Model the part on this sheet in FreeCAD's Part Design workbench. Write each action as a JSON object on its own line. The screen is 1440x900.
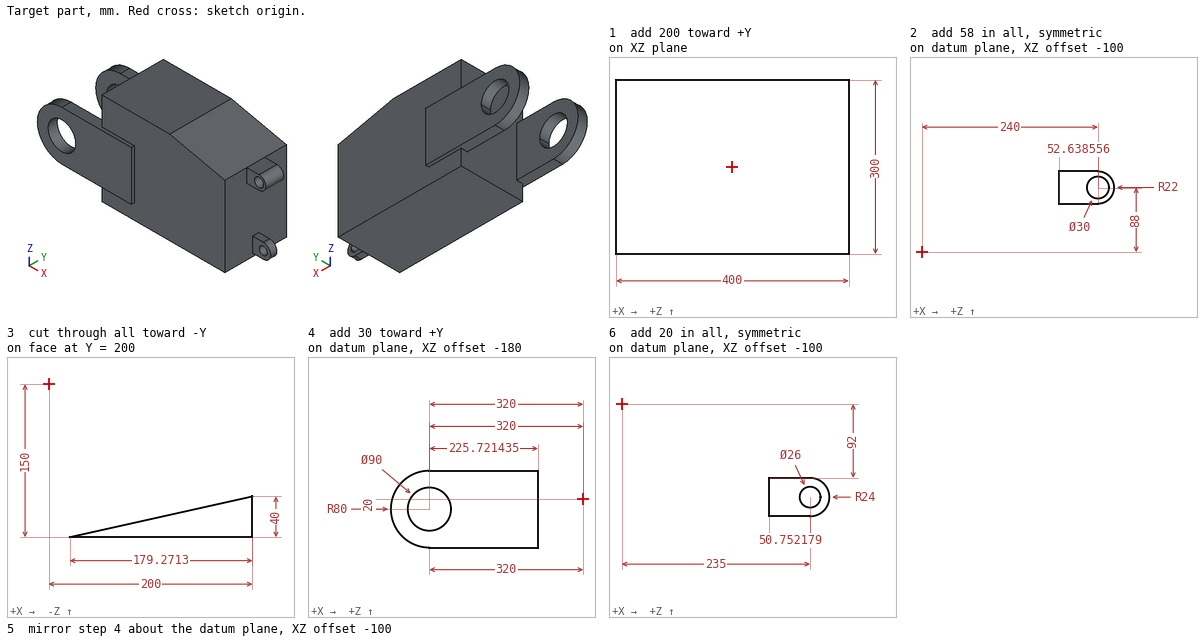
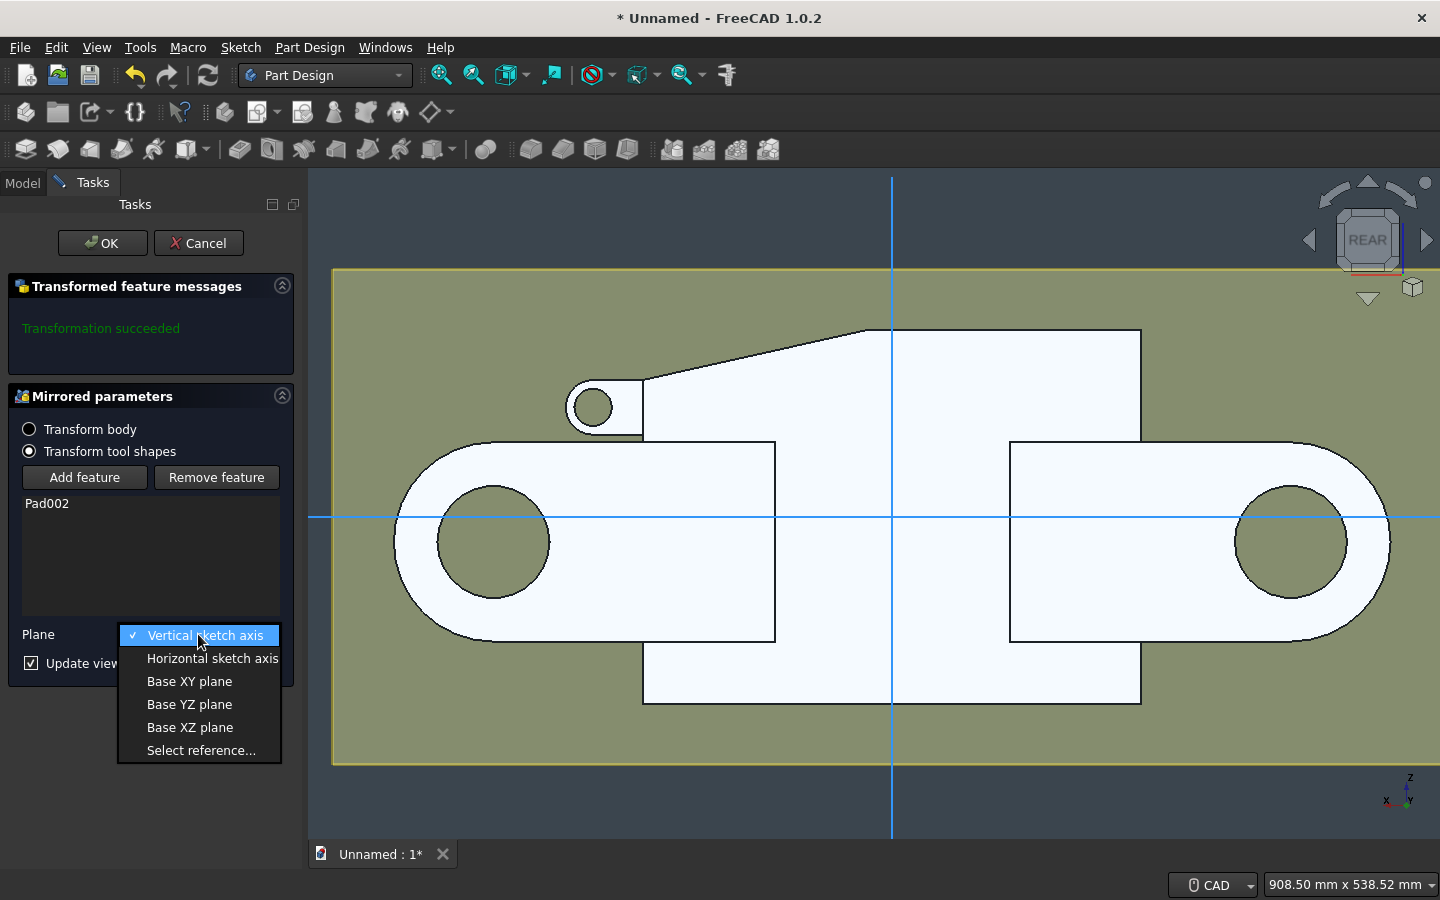
{"action": "left_click", "coordinate": [198, 750]}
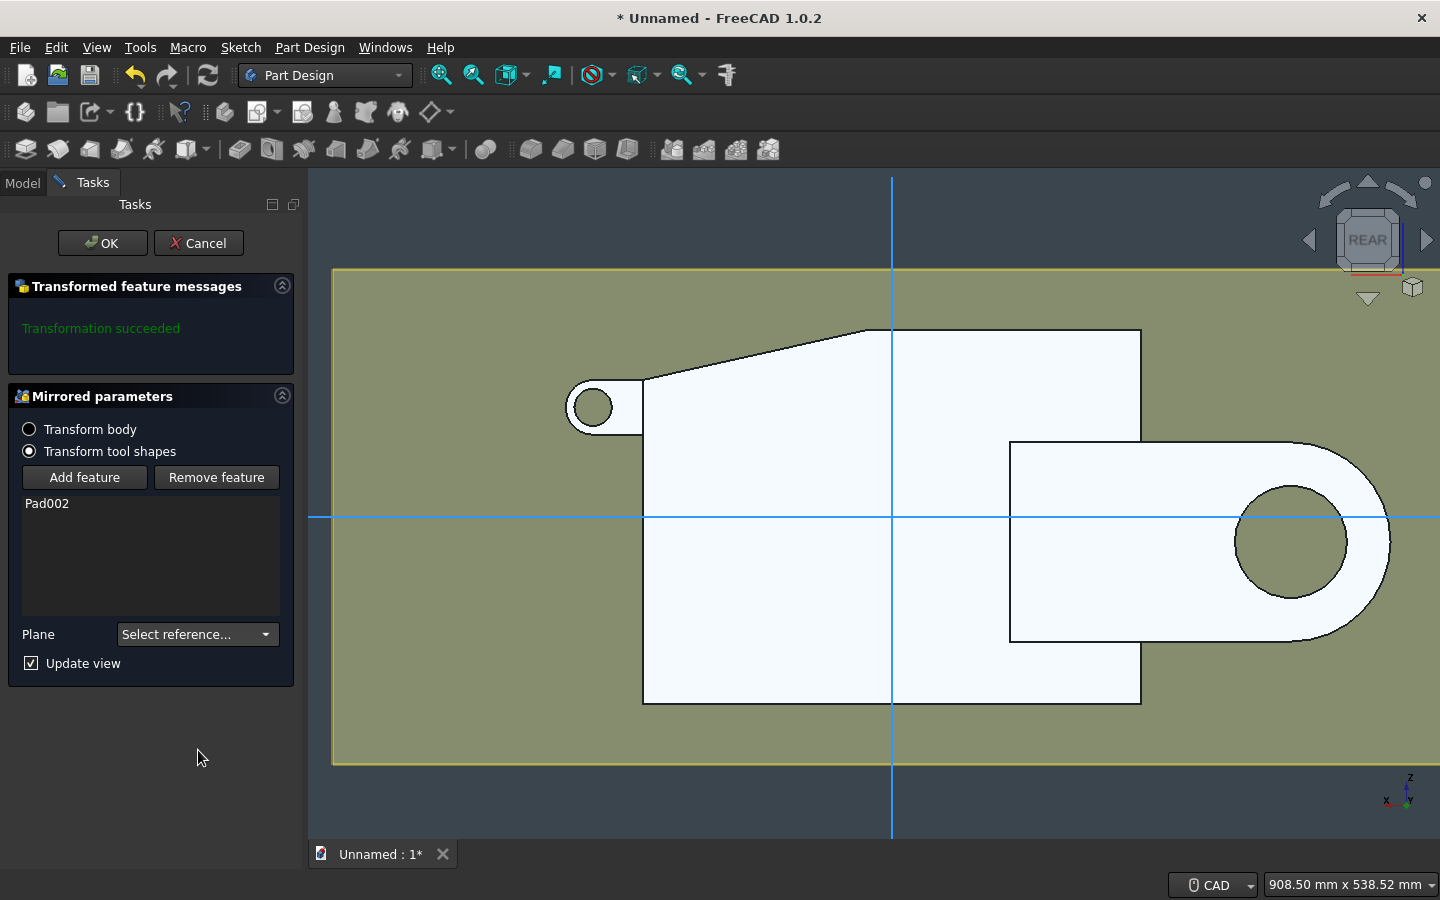
{"action": "left_click", "coordinate": [23, 182]}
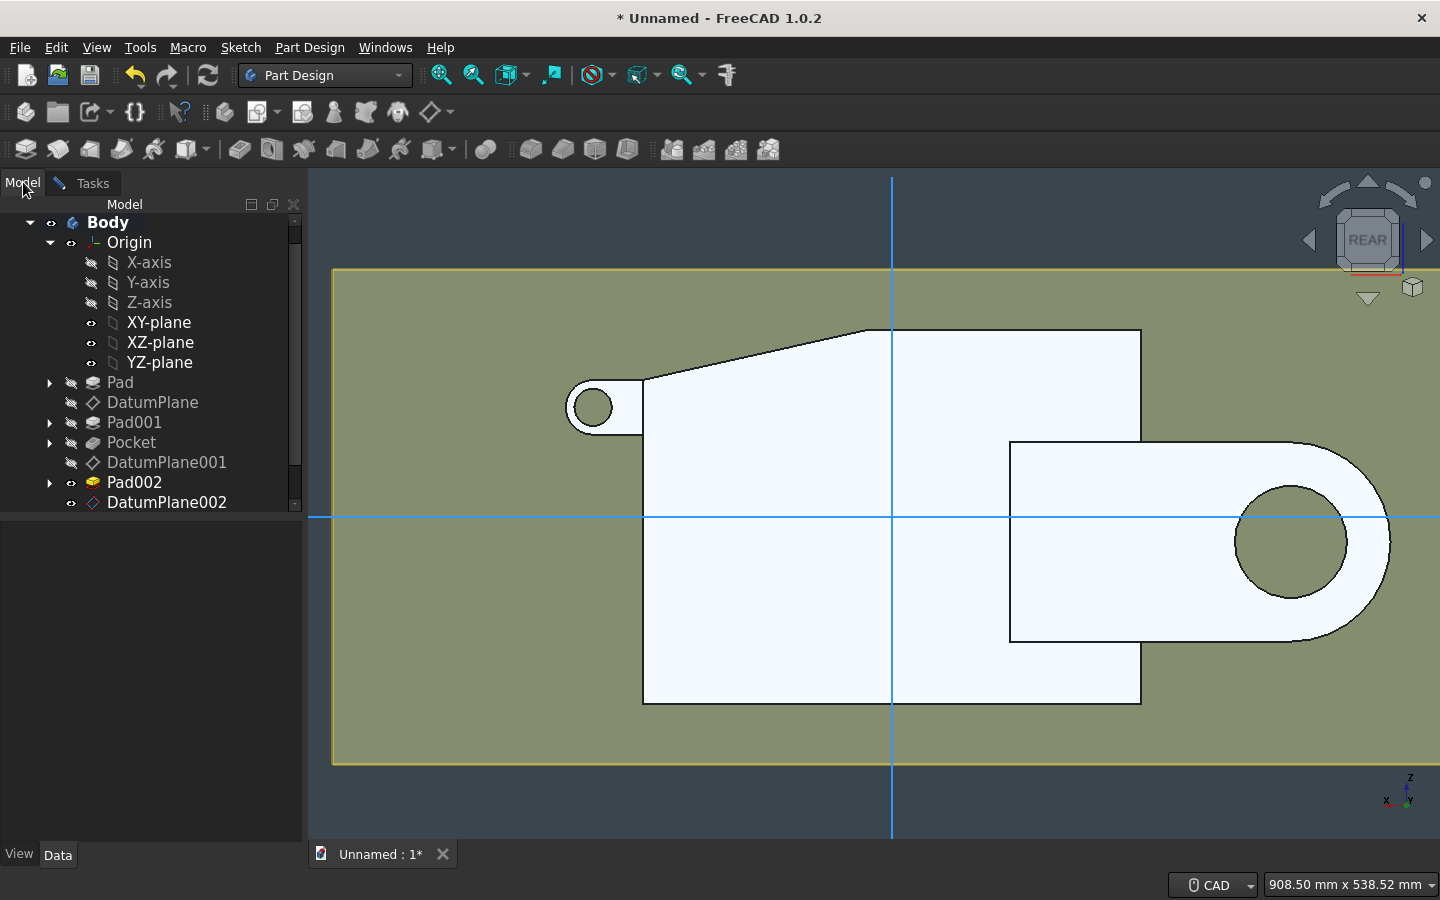
{"action": "left_click", "coordinate": [116, 503]}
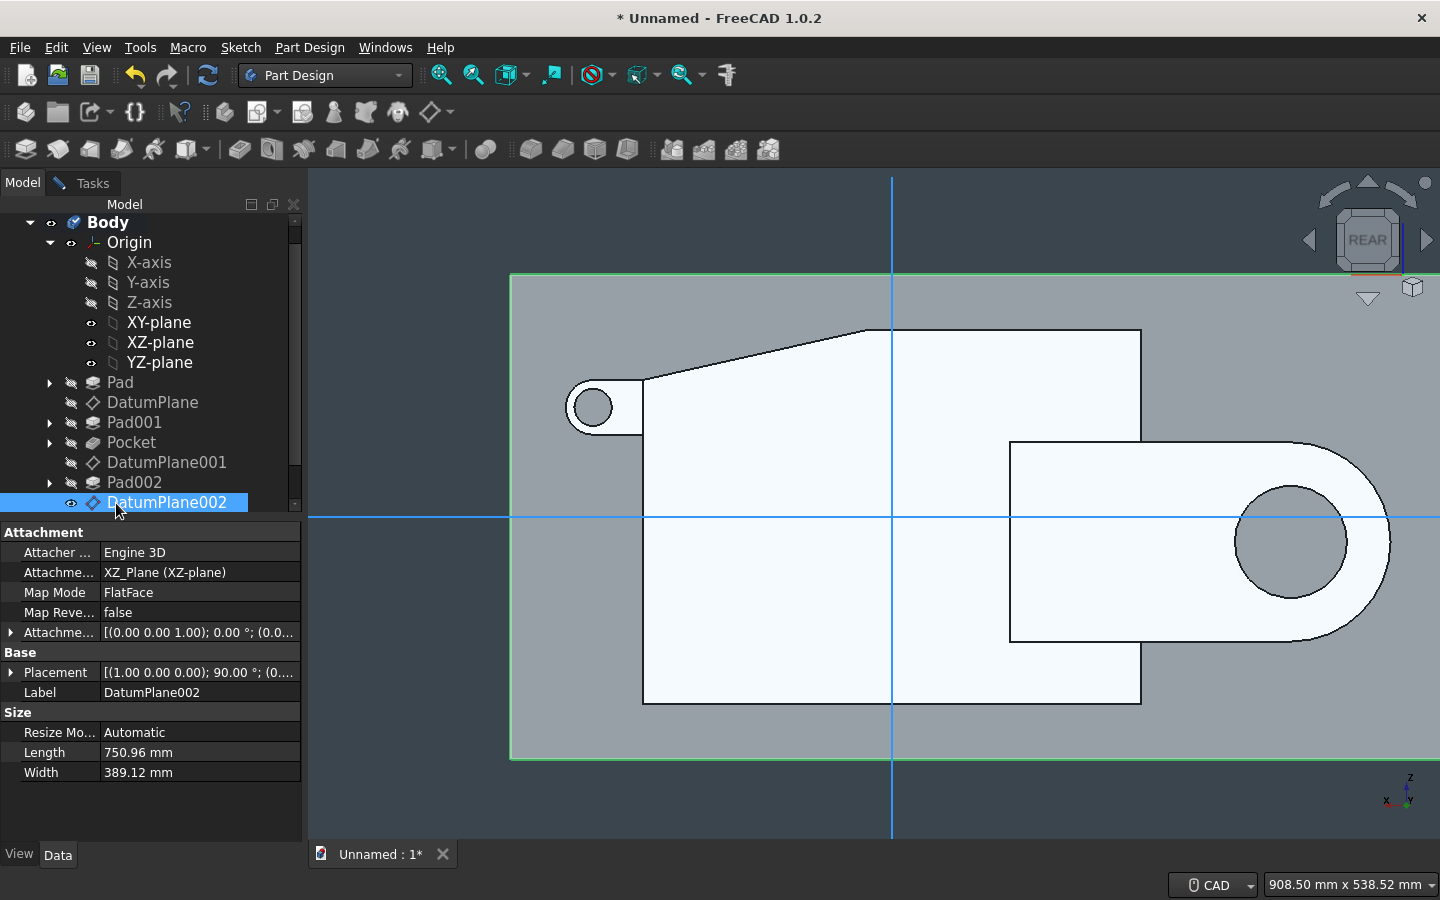
{"action": "left_click", "coordinate": [84, 182]}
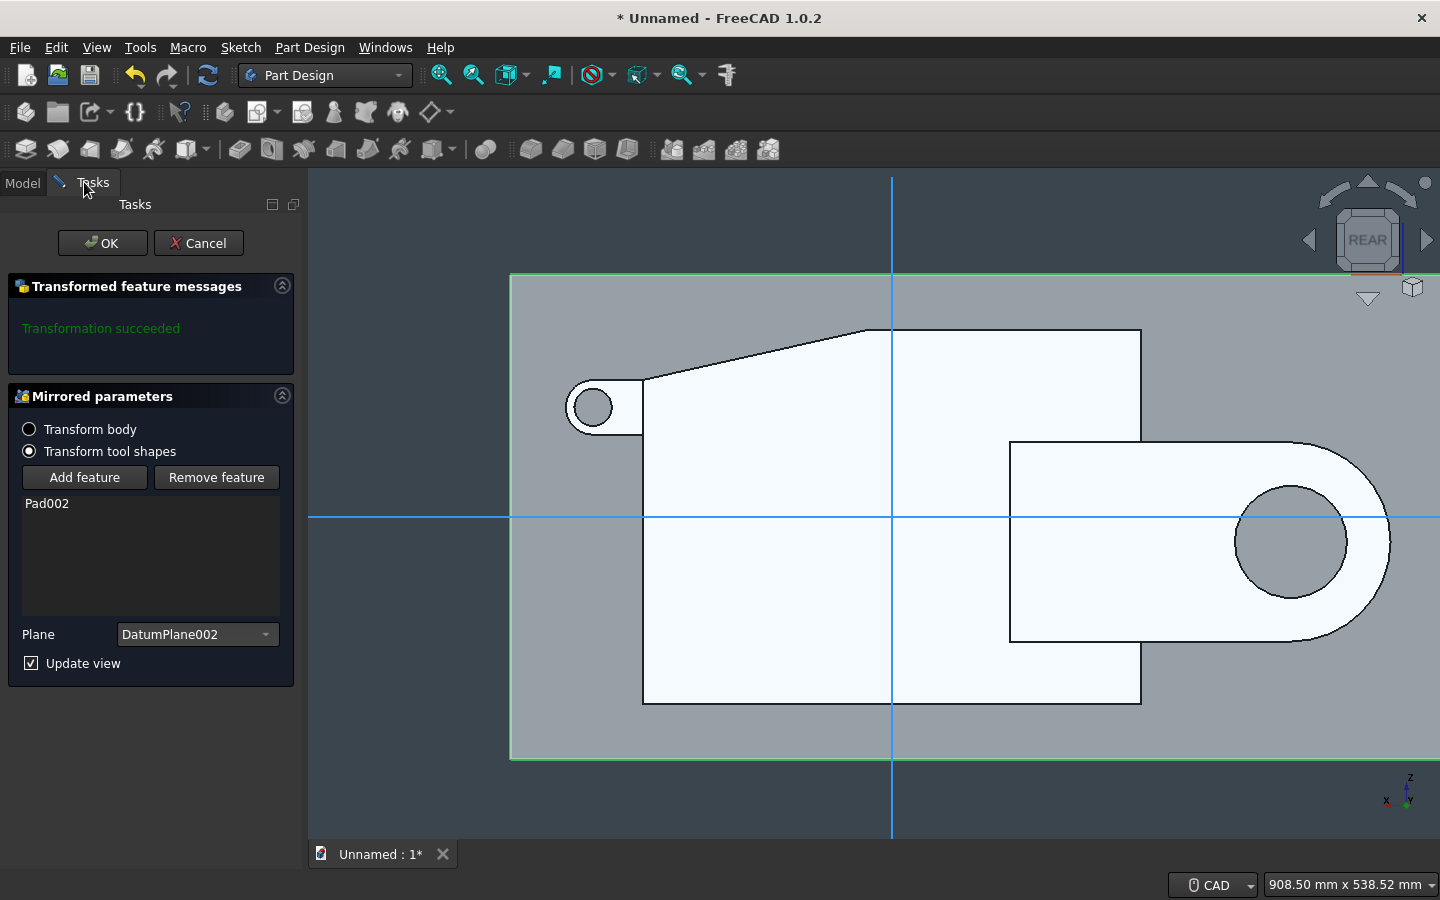
{"action": "left_click", "coordinate": [103, 243]}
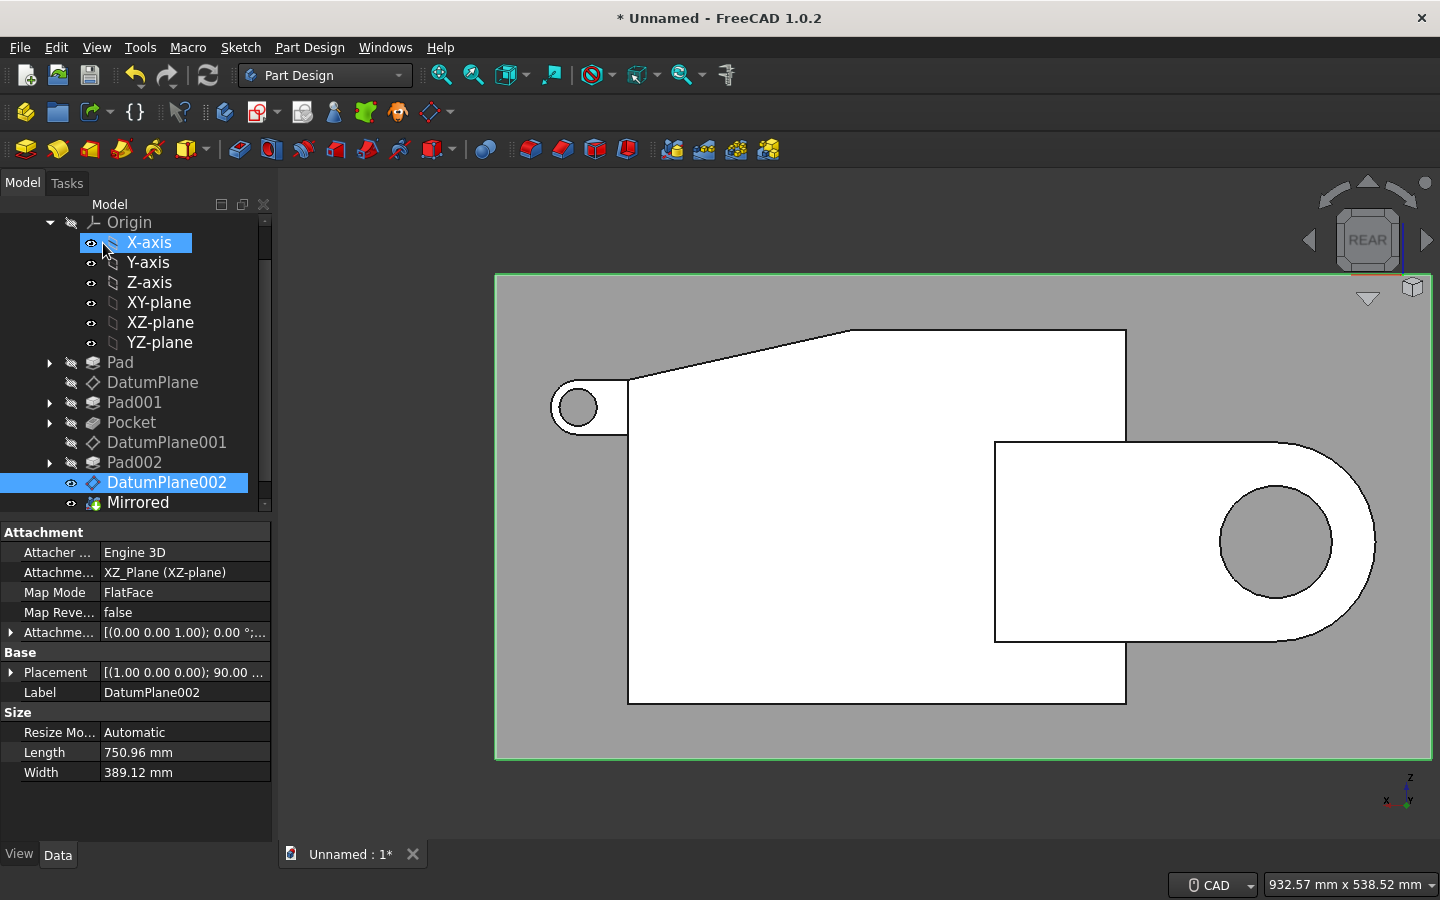
{"action": "left_click", "coordinate": [116, 483]}
{"action": "key", "text": "space"}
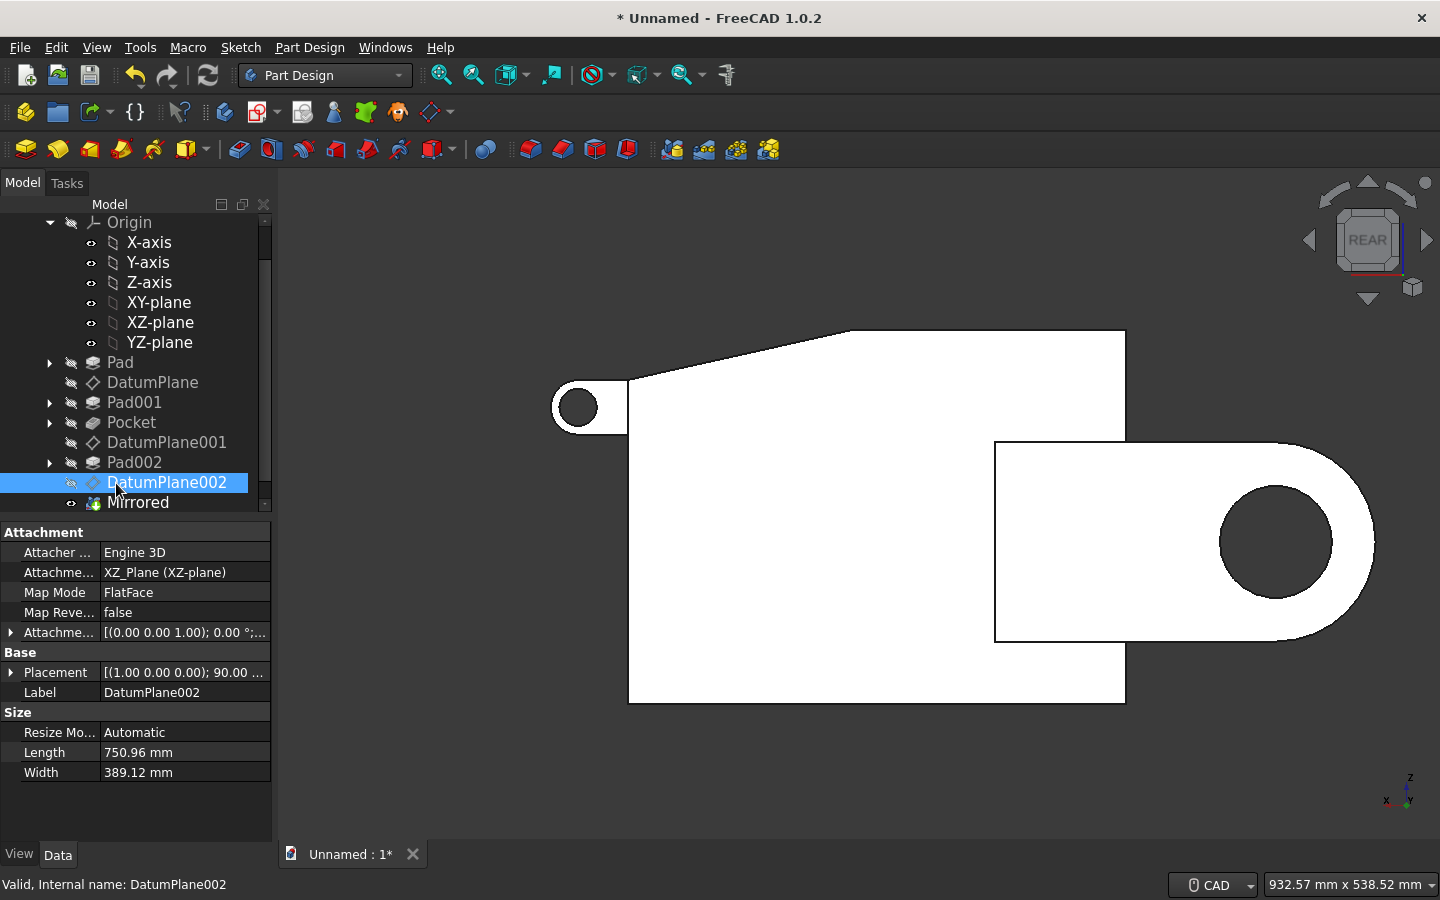
{"action": "left_click", "coordinate": [136, 323]}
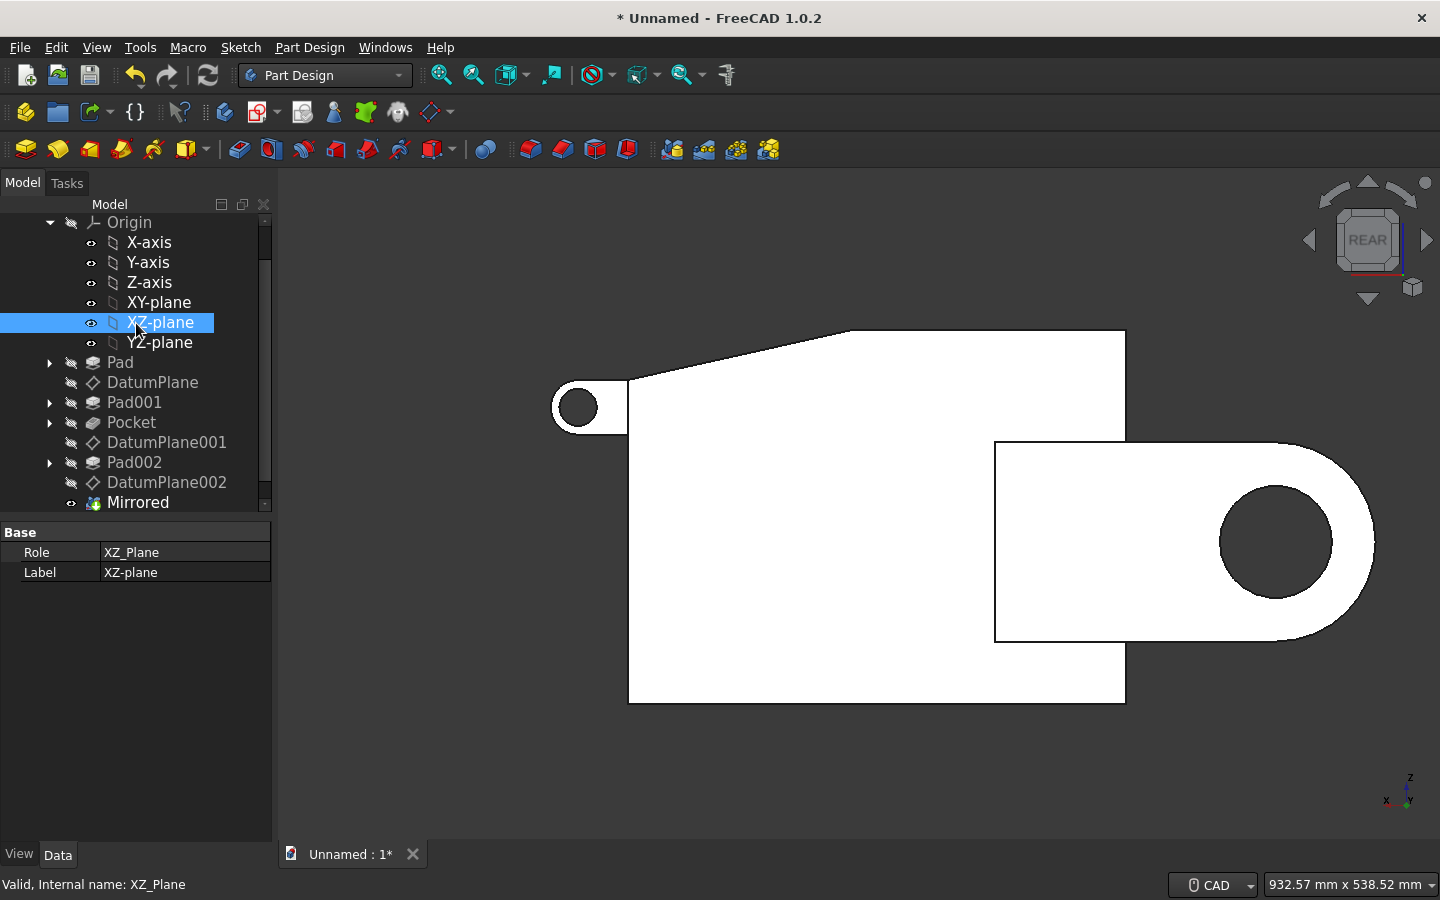
{"action": "left_click", "coordinate": [430, 112]}